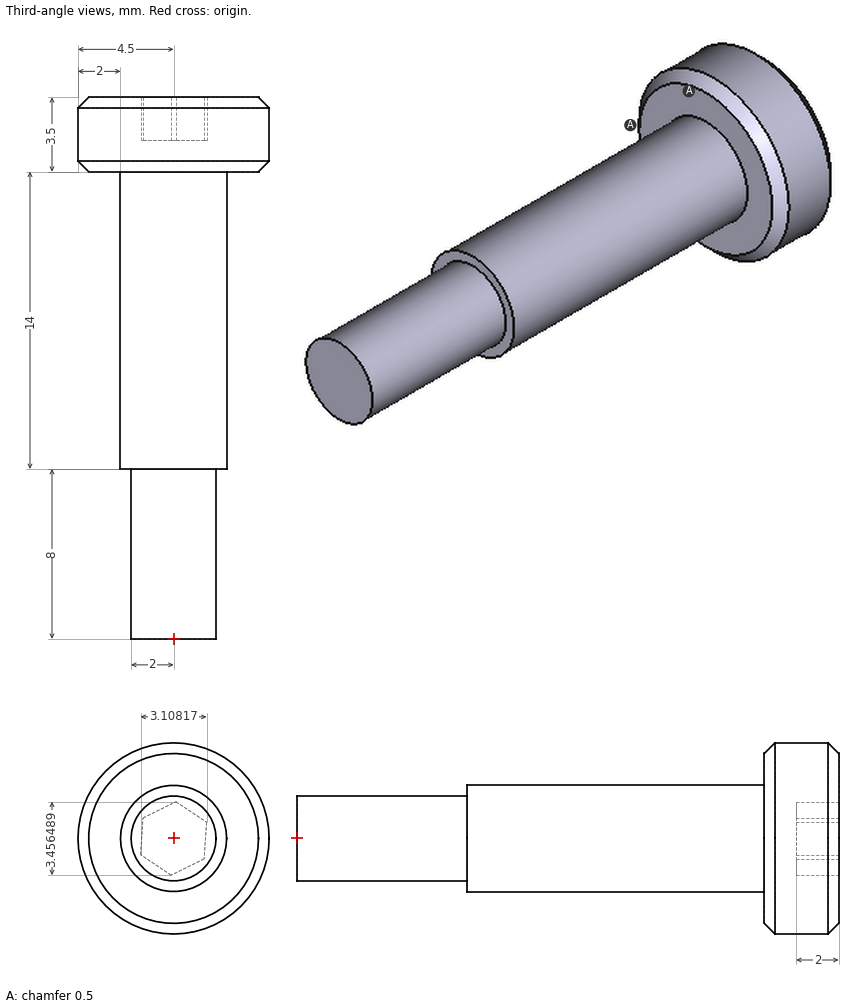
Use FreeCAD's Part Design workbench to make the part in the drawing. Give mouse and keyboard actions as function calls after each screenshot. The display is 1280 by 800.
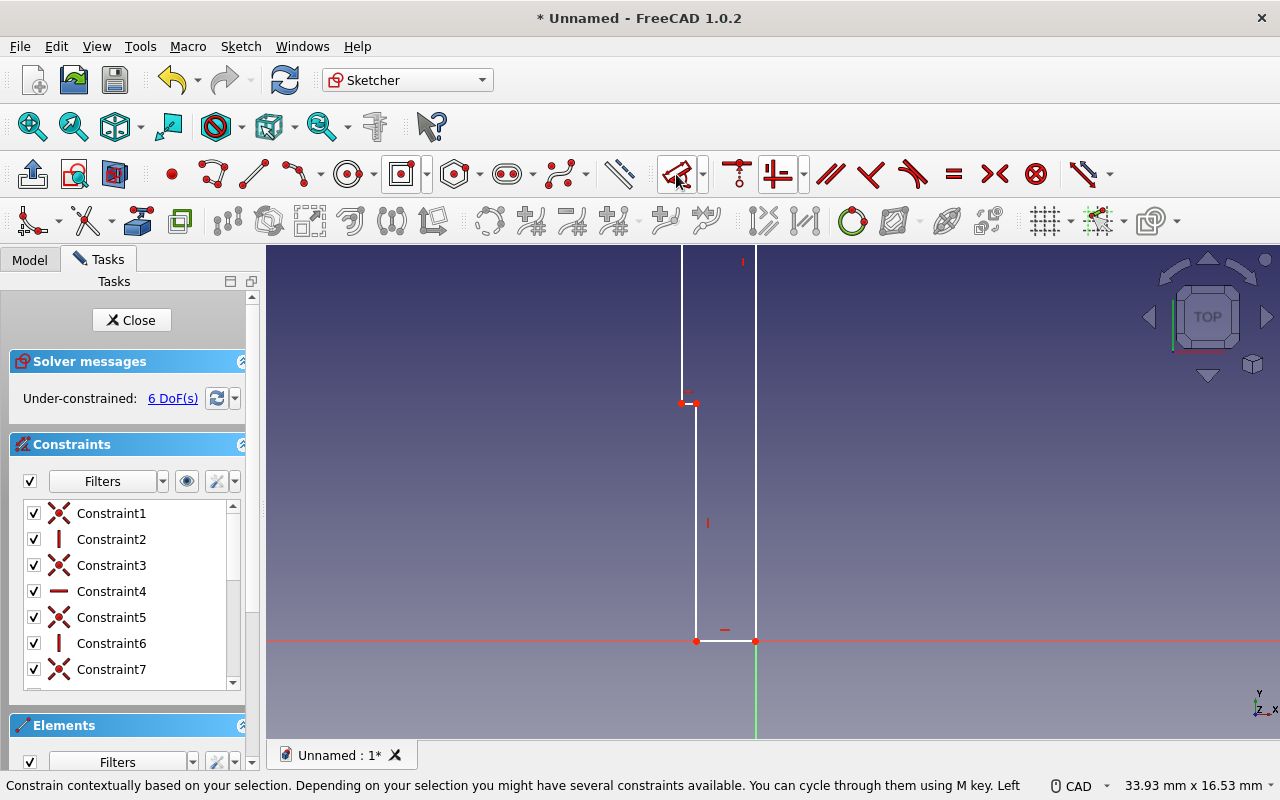
scroll(714, 627, down, 5)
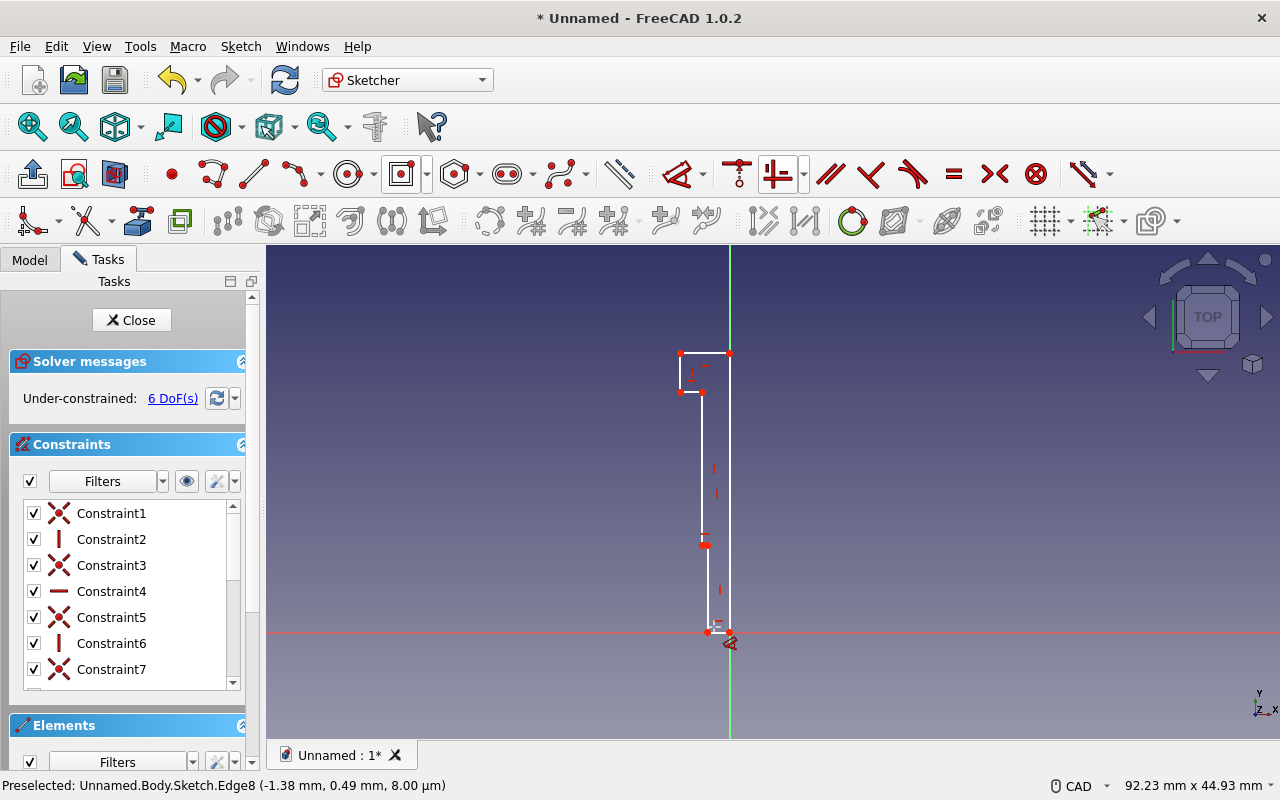
scroll(687, 392, up, 4)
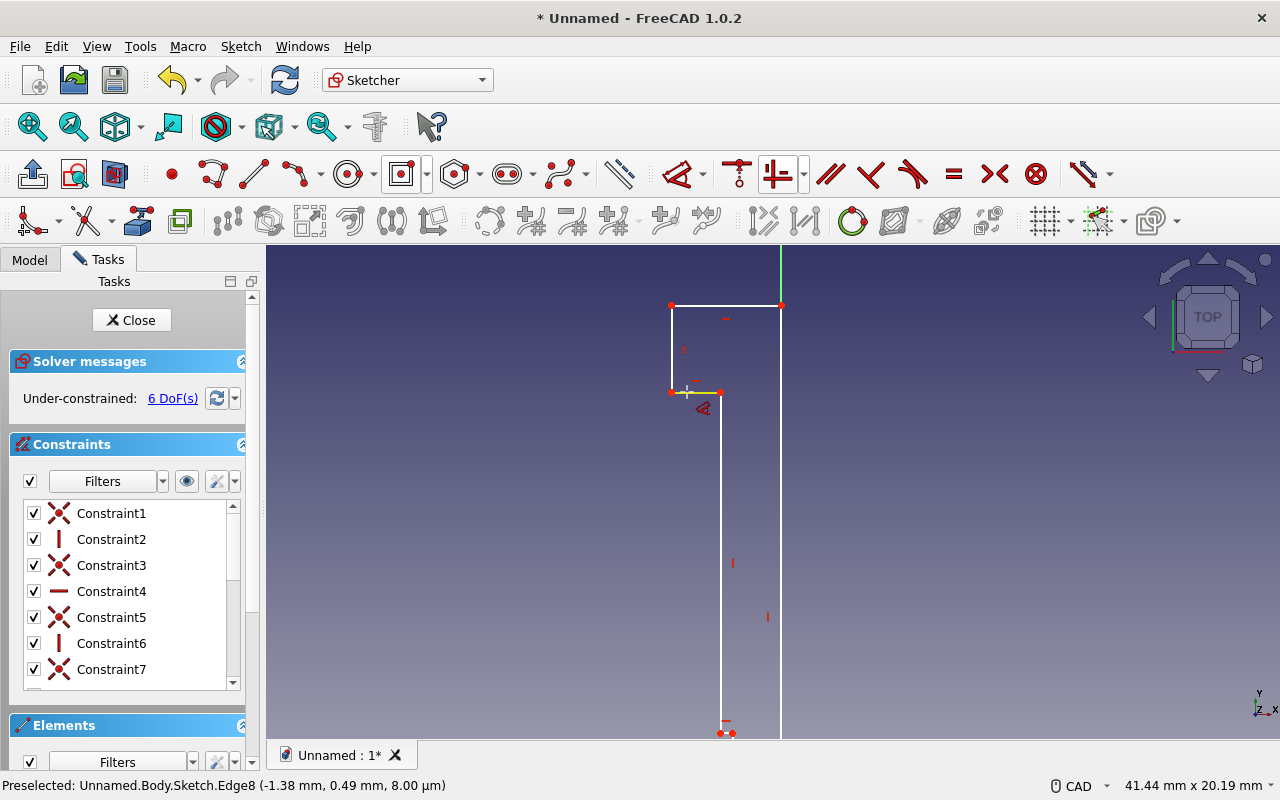
click(686, 393)
click(696, 359)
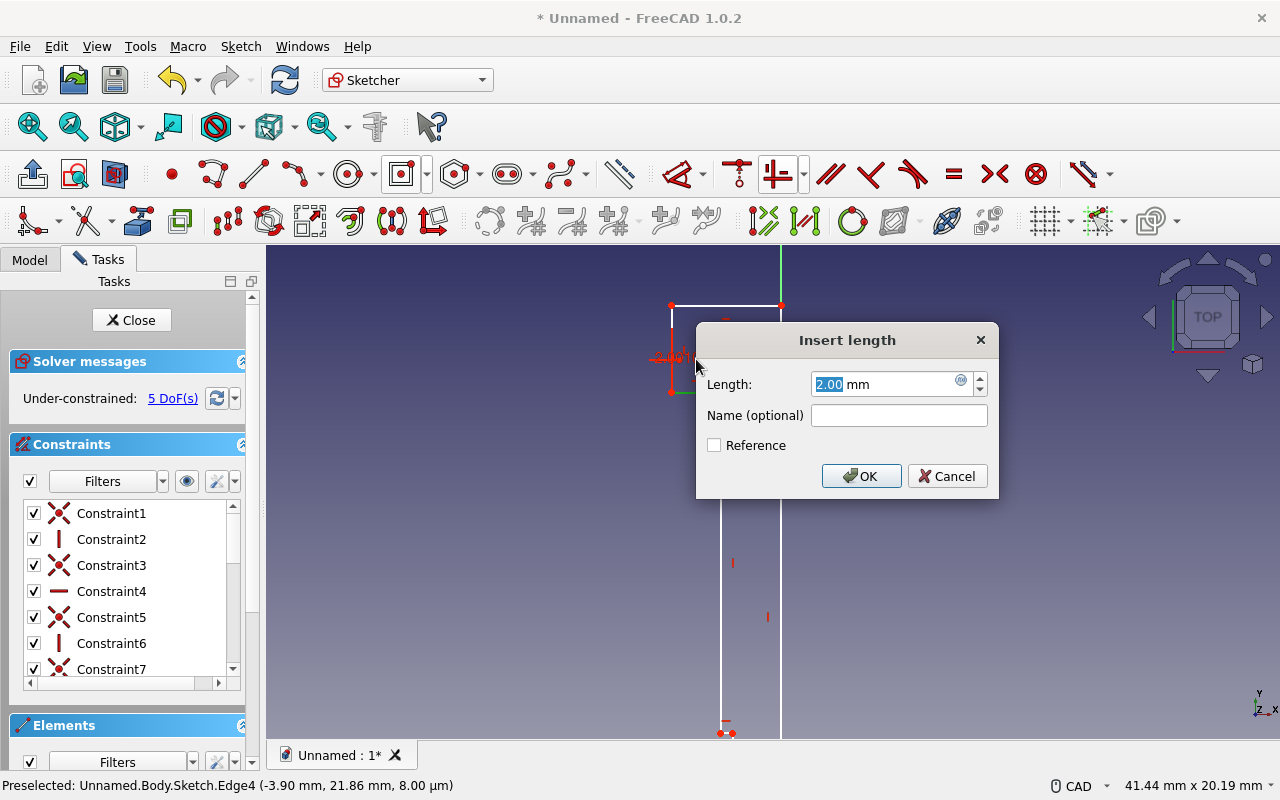
text(2)
key(Return)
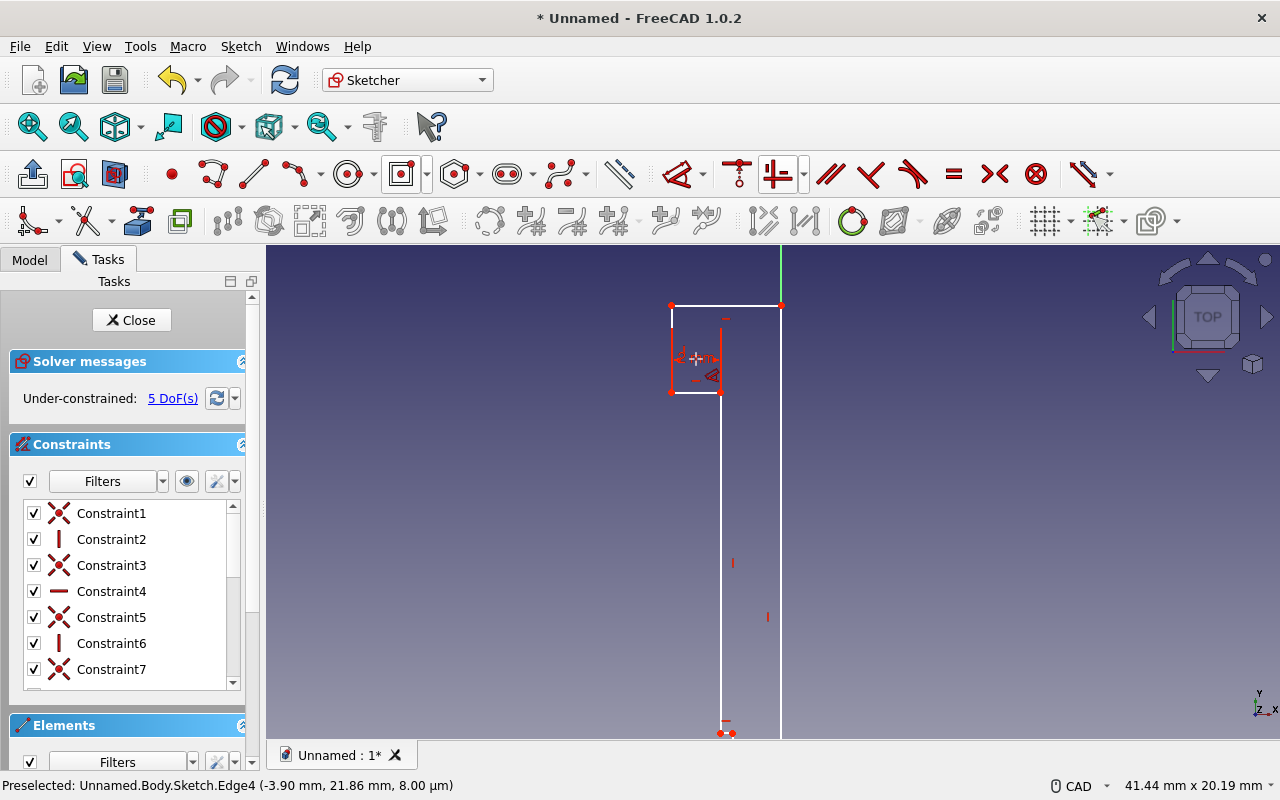
scroll(687, 391, down, 4)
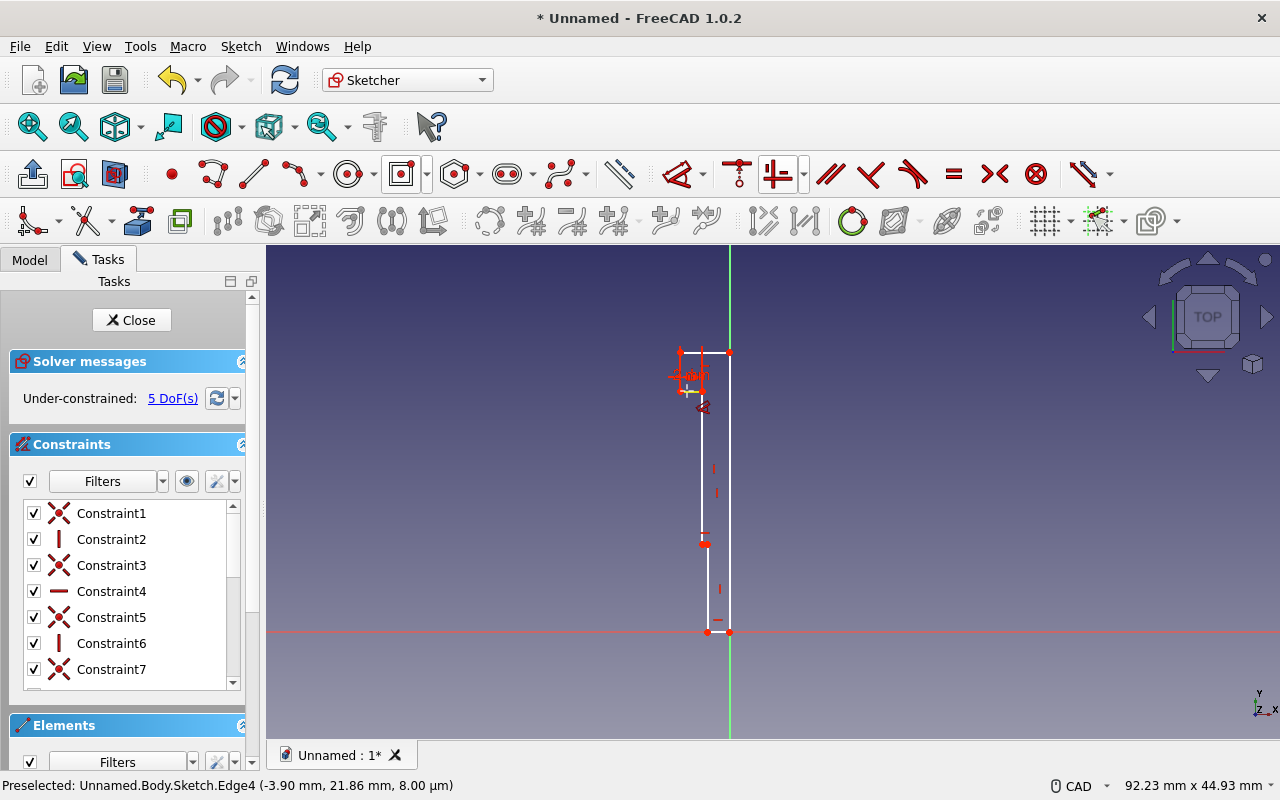
click(708, 571)
click(674, 589)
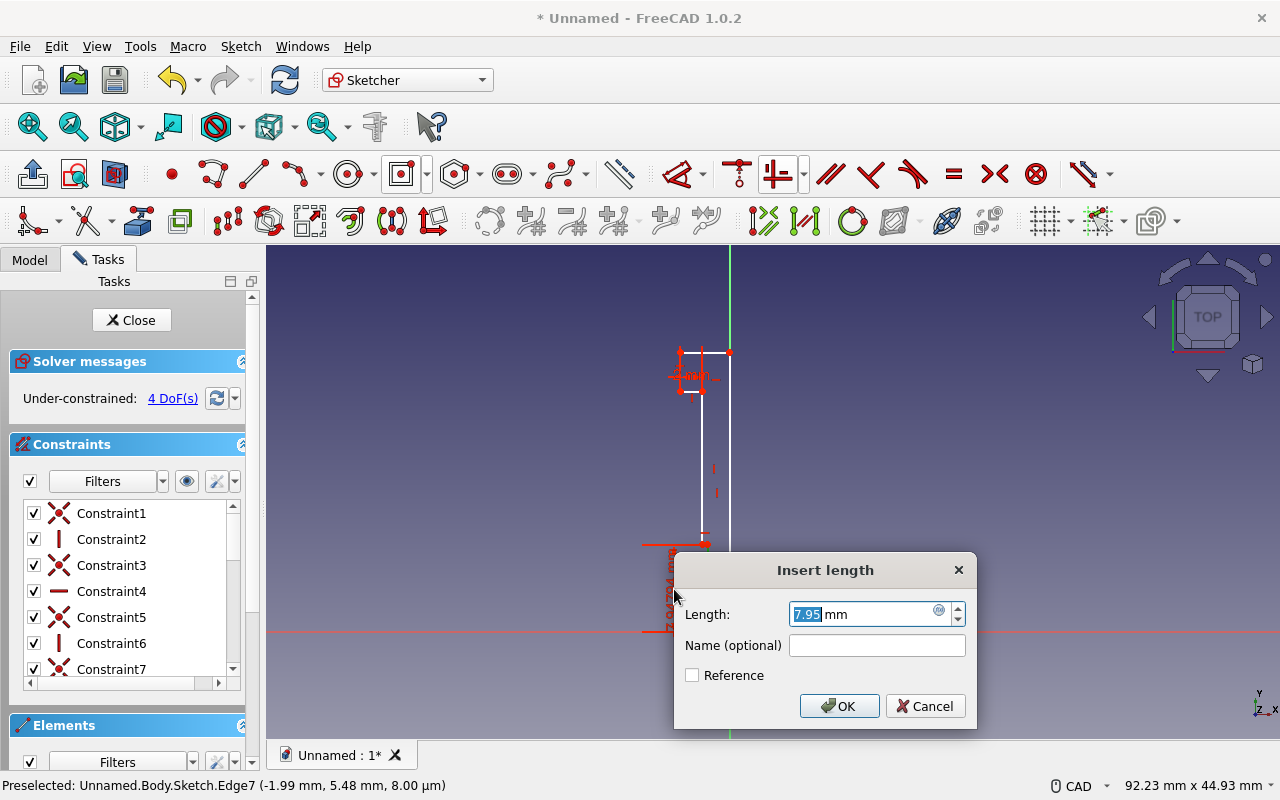
text(8)
key(Return)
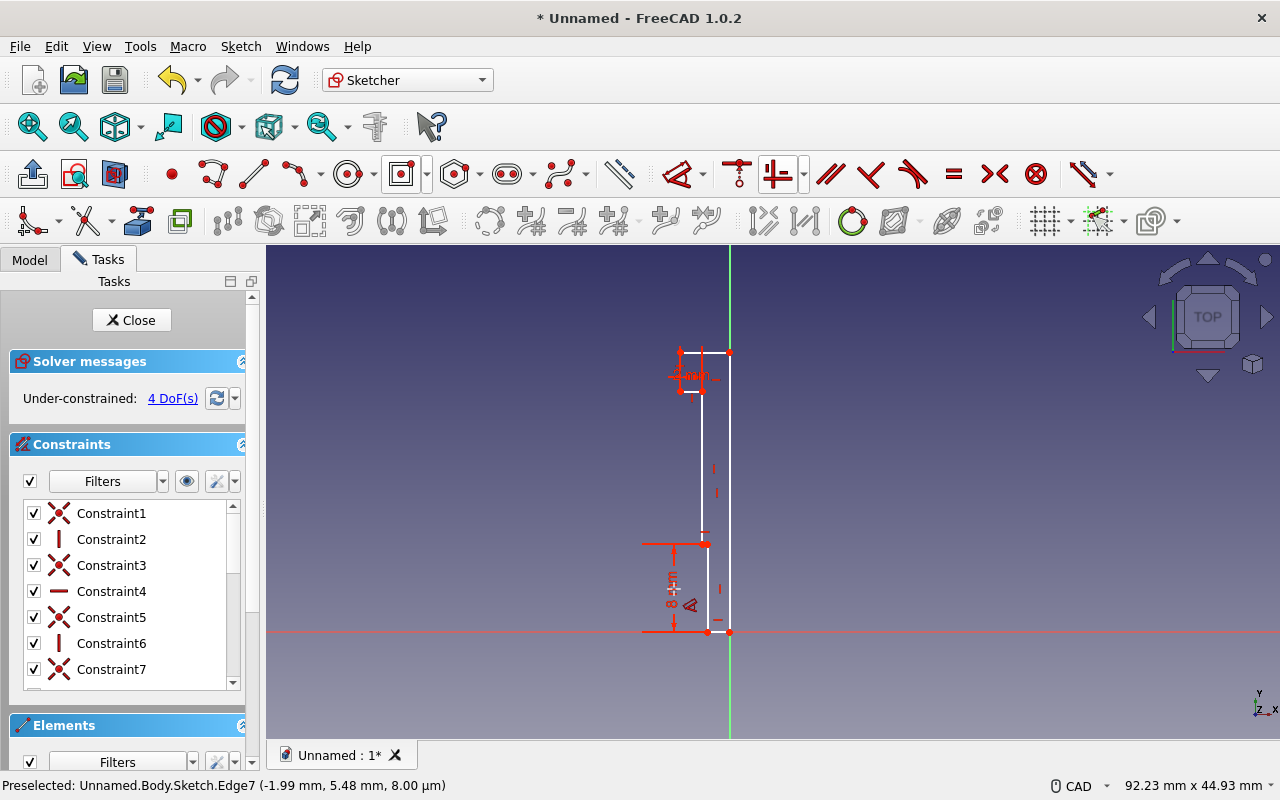
scroll(719, 632, up, 3)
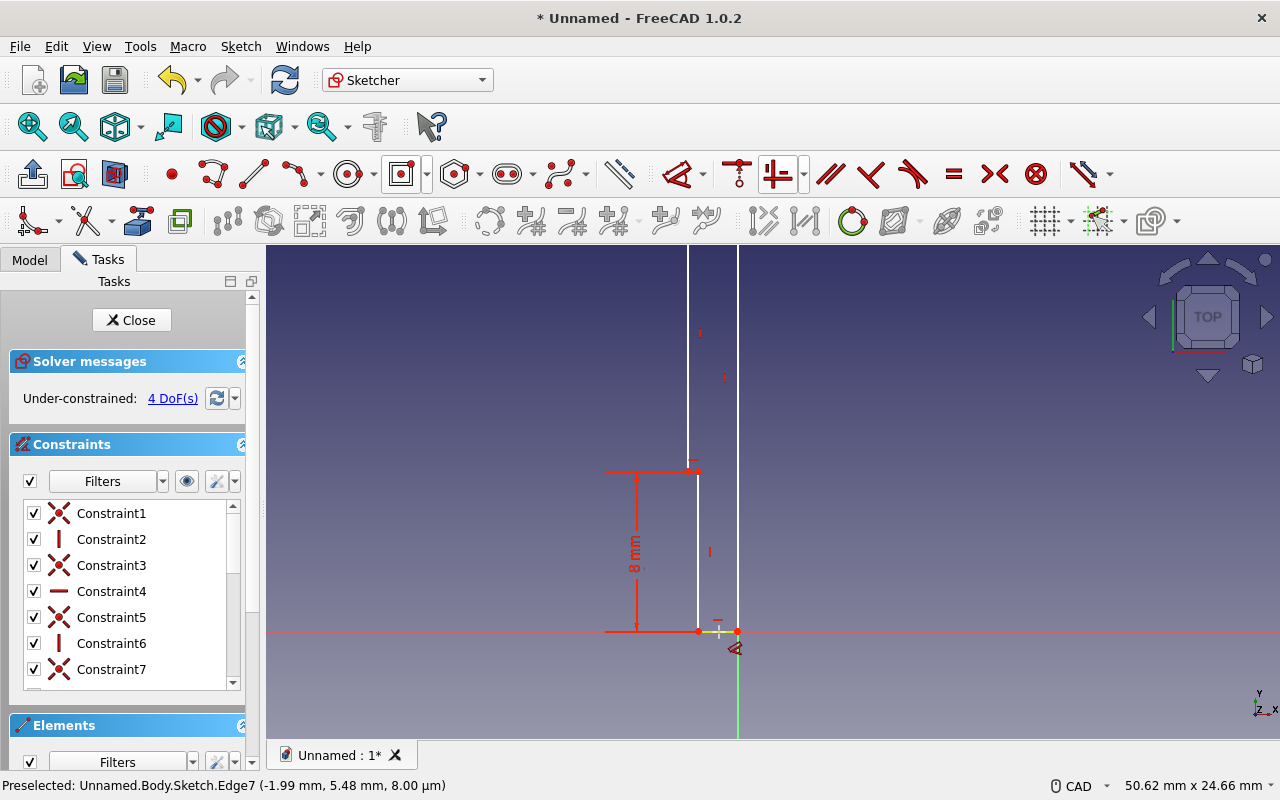
click(718, 632)
click(718, 666)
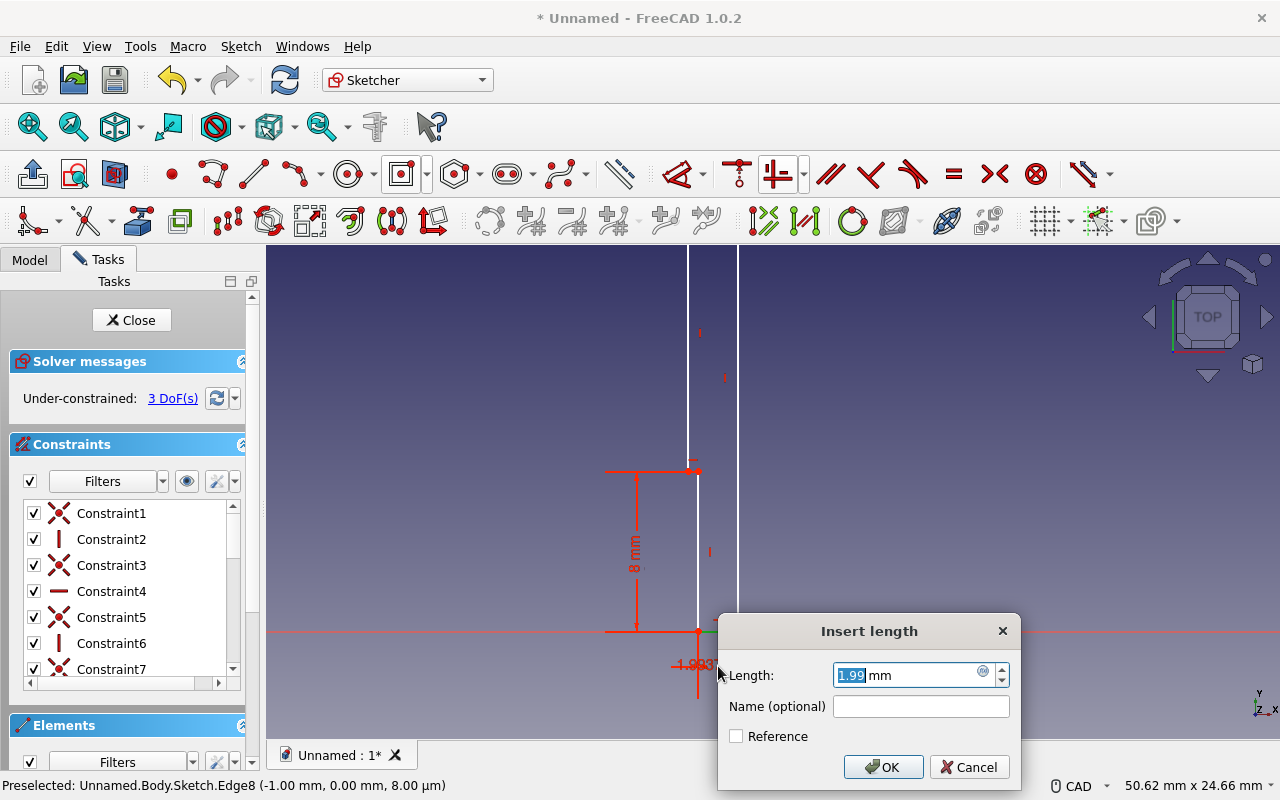
text(2)
key(Return)